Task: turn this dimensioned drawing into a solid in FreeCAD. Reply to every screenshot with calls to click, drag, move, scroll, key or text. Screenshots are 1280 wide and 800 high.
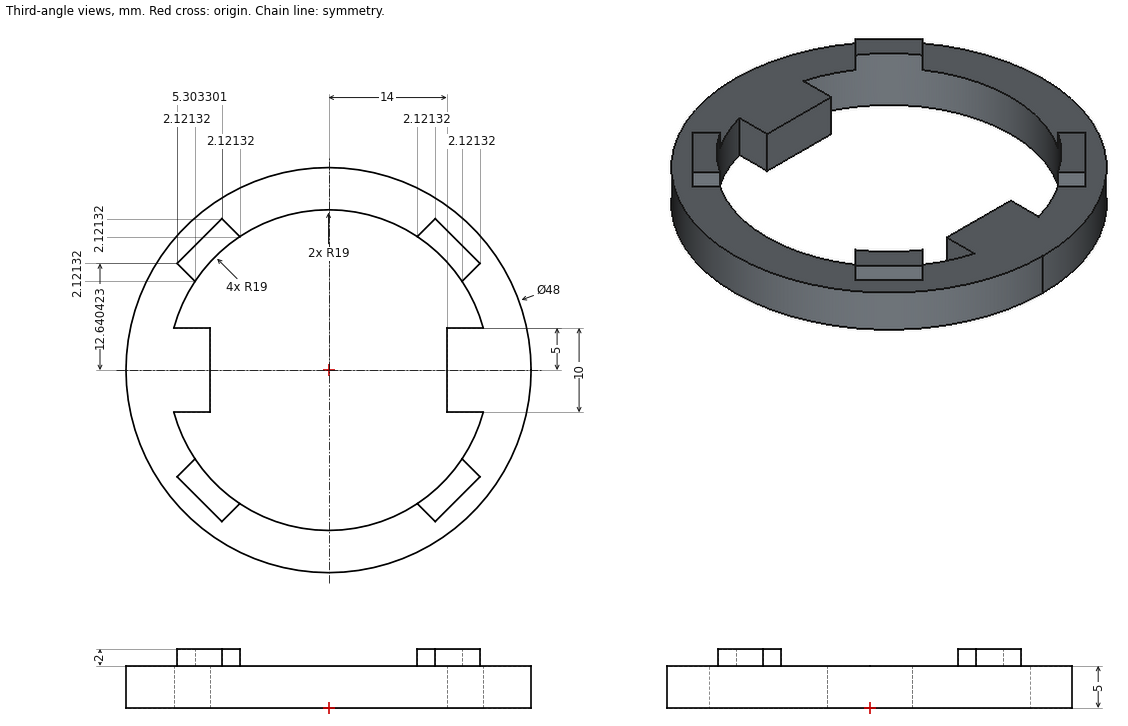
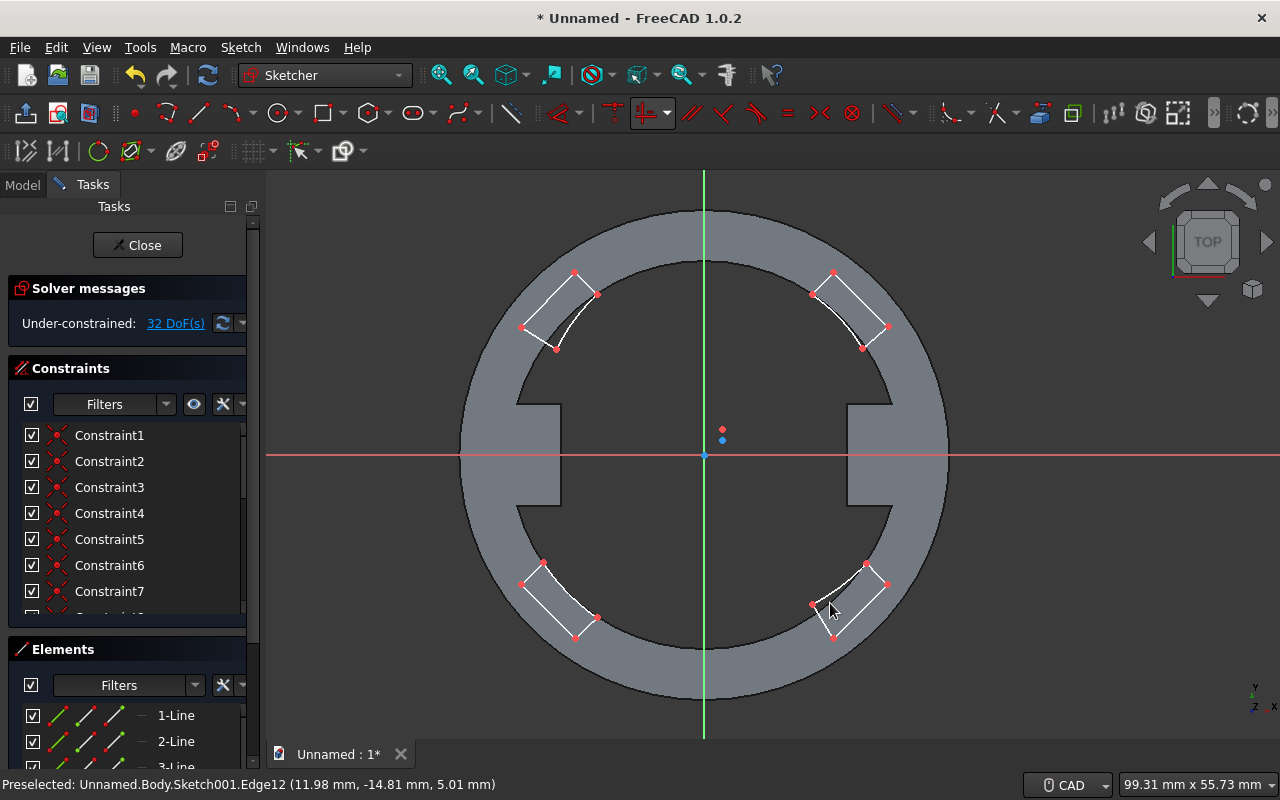
click(583, 309)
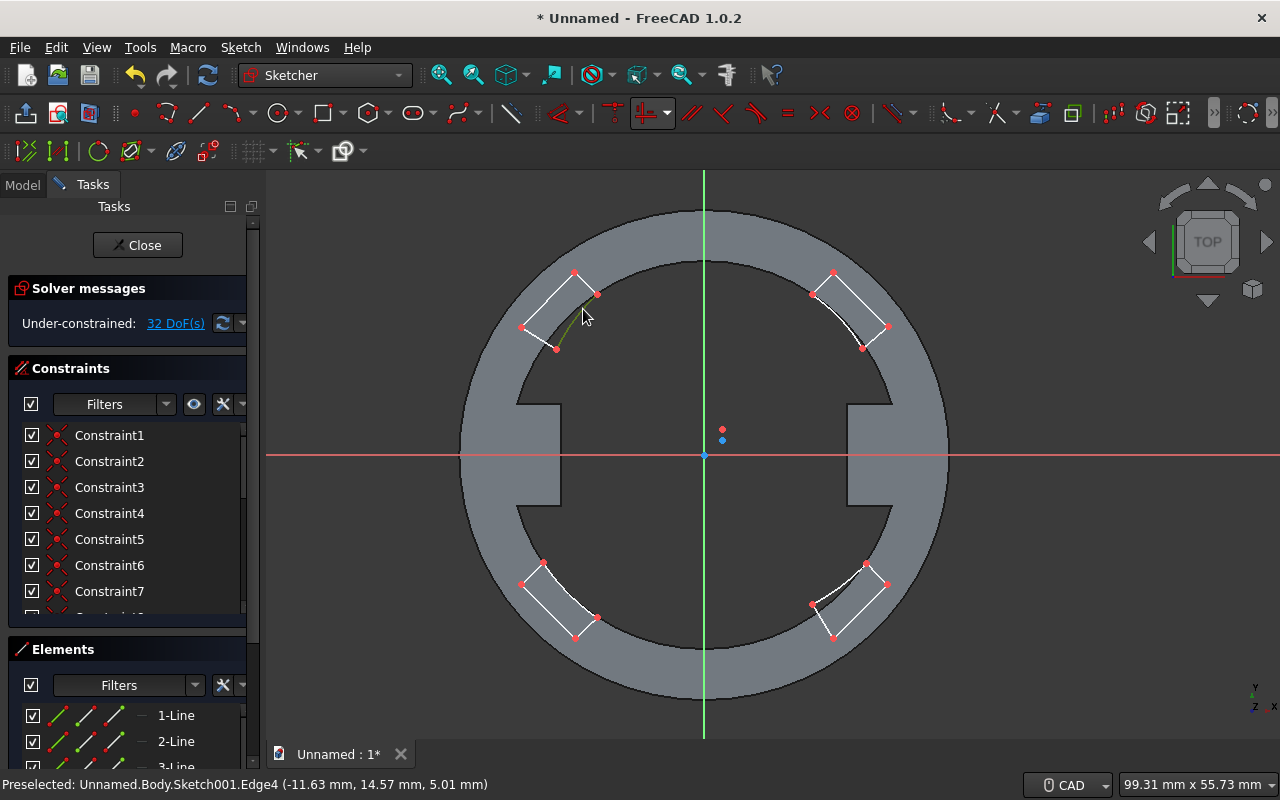
click(557, 581)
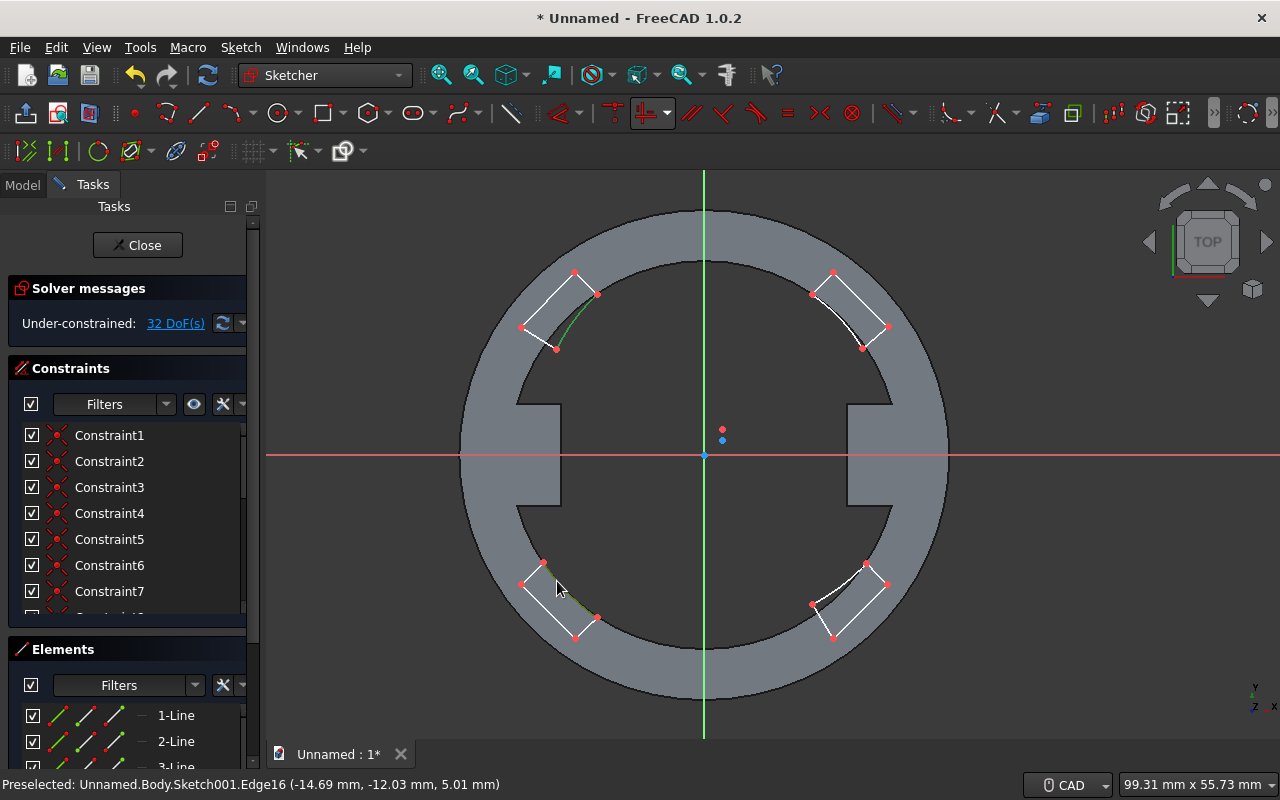
key(c)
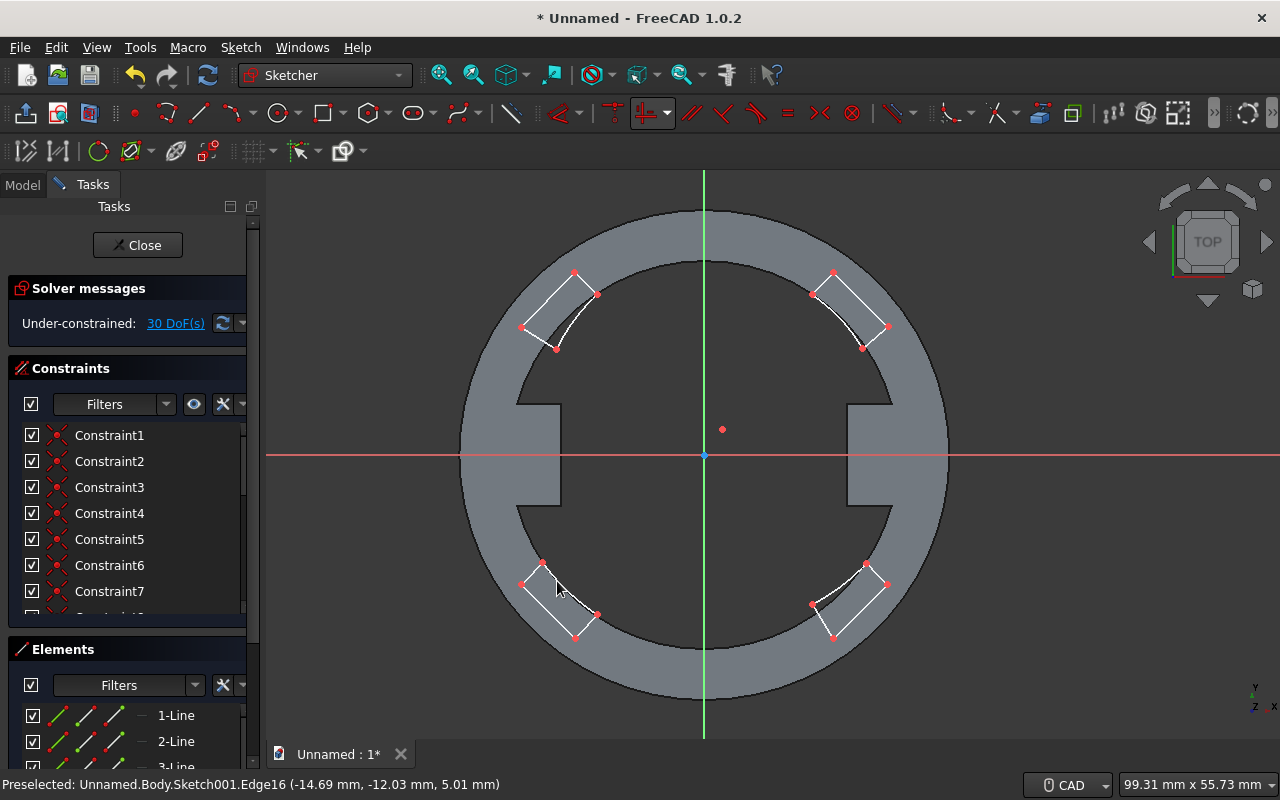
drag(694, 420, 732, 465)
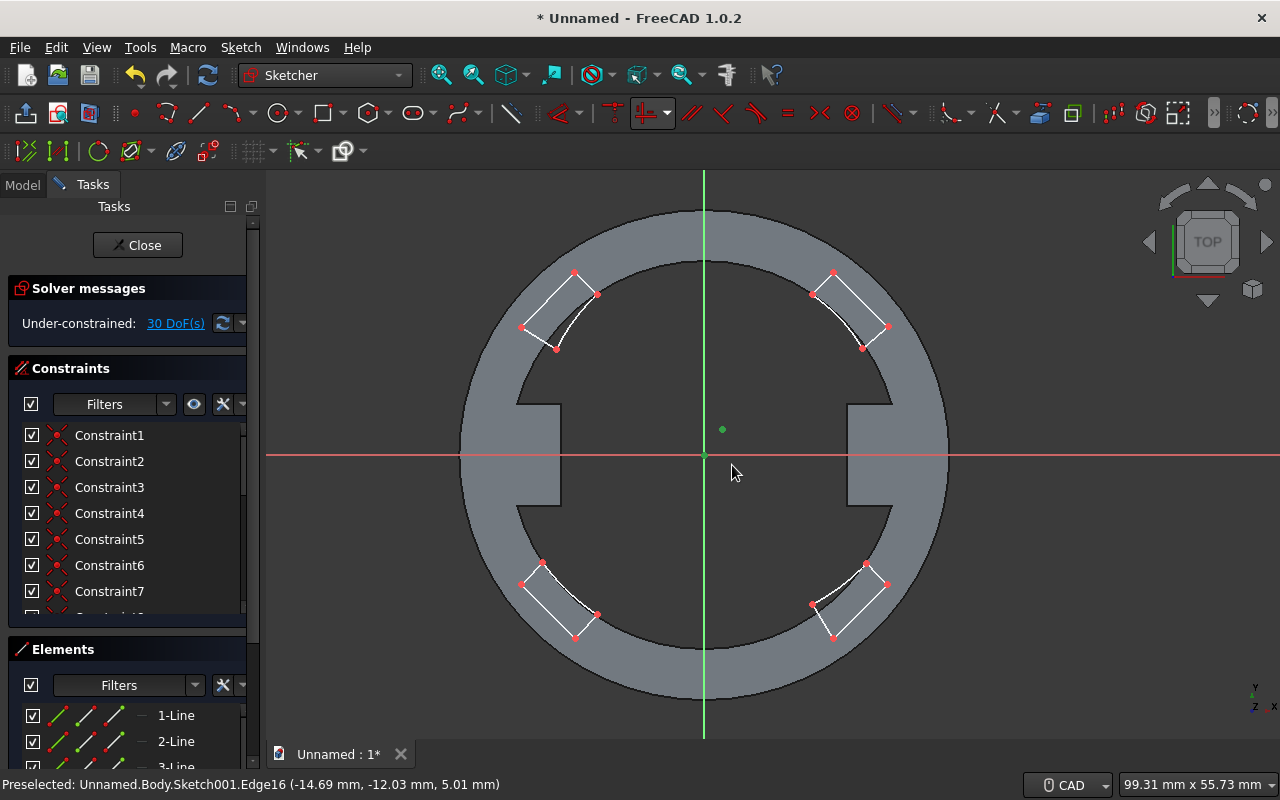
click(614, 114)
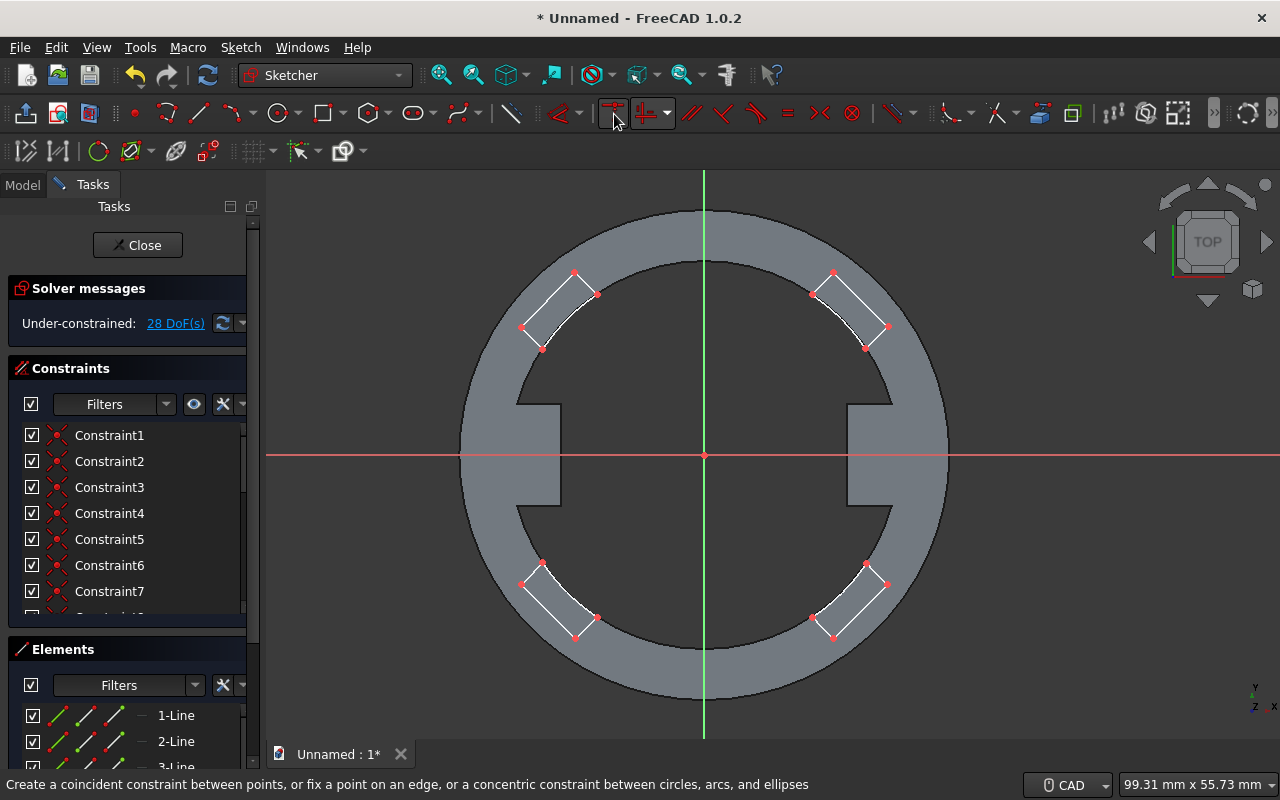
click(579, 309)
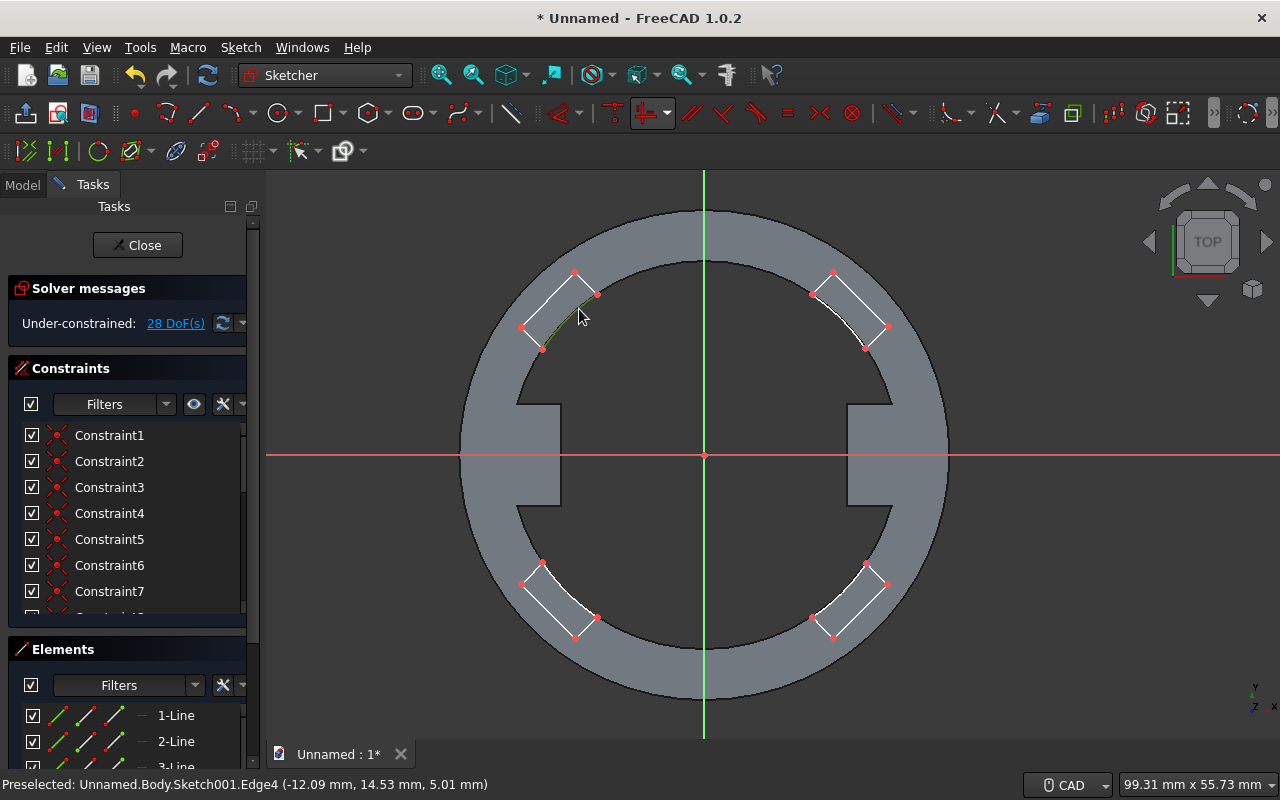
click(852, 331)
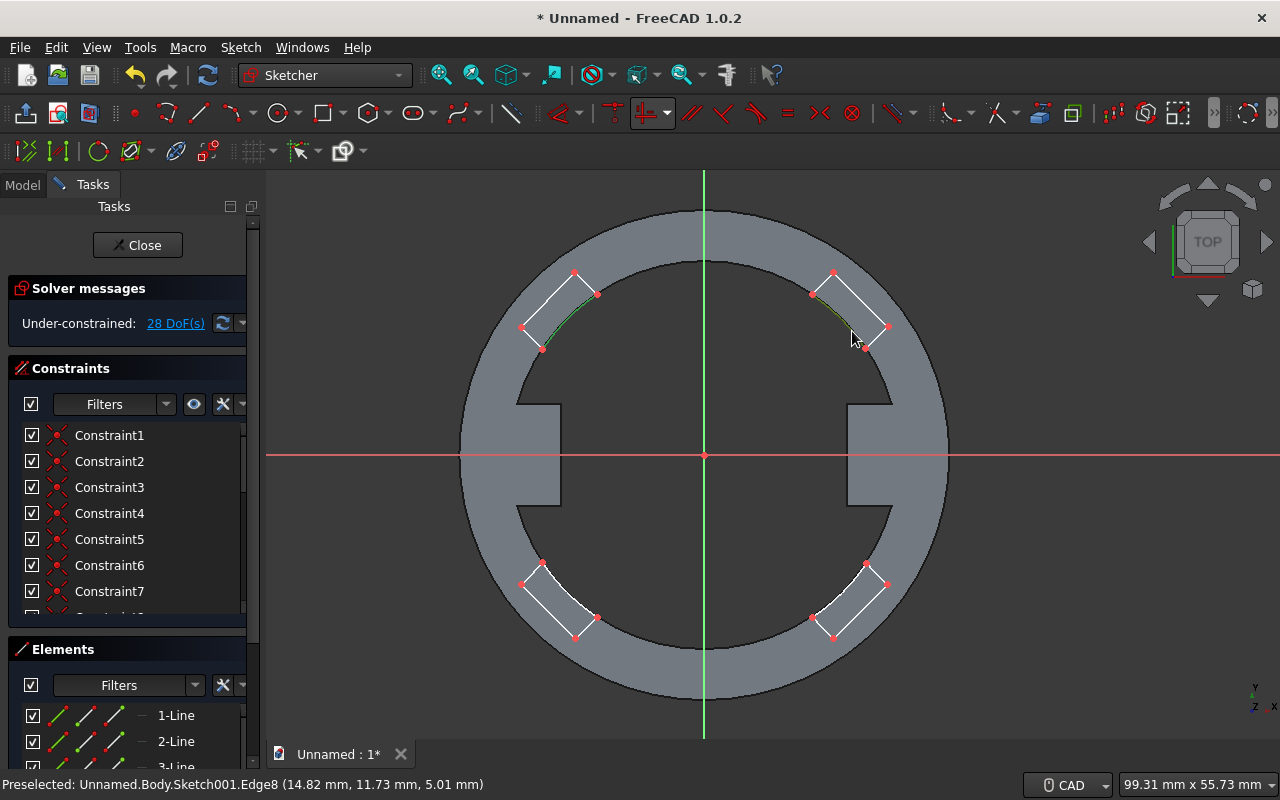
click(831, 603)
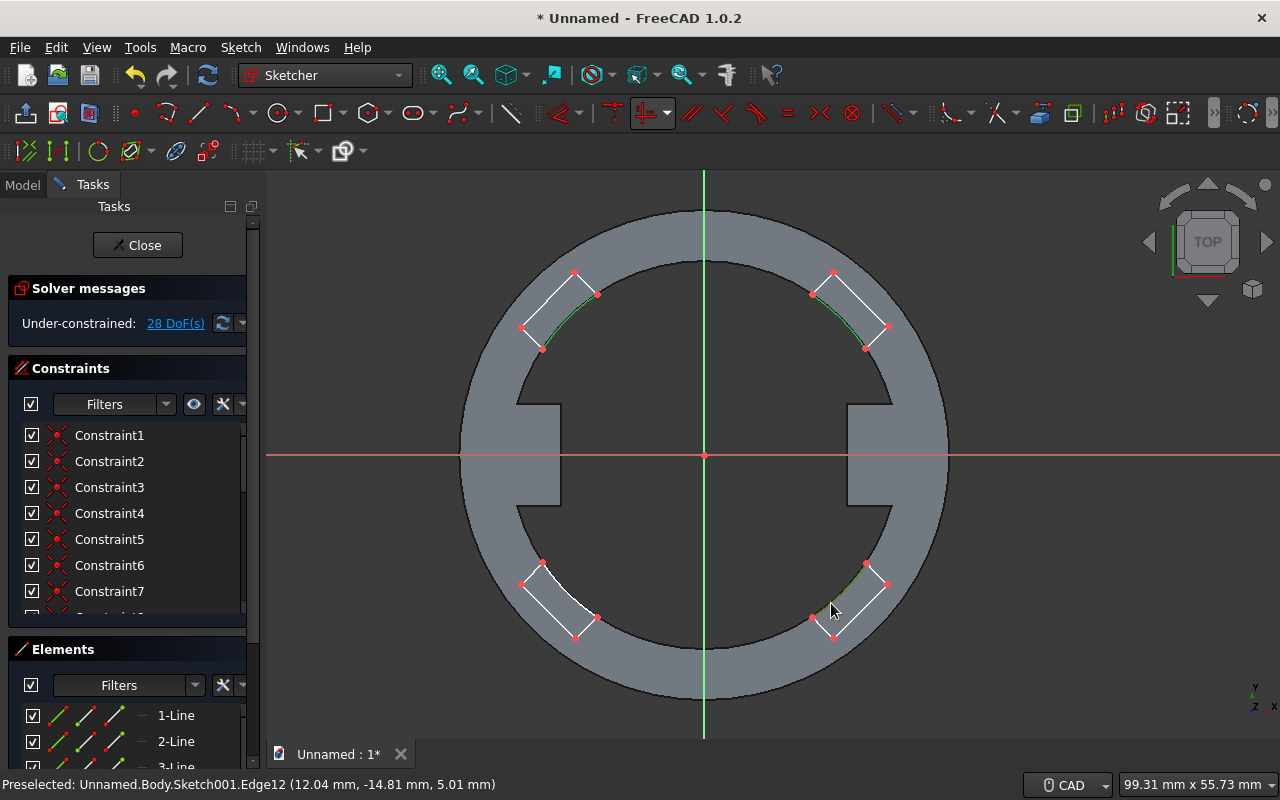
click(557, 581)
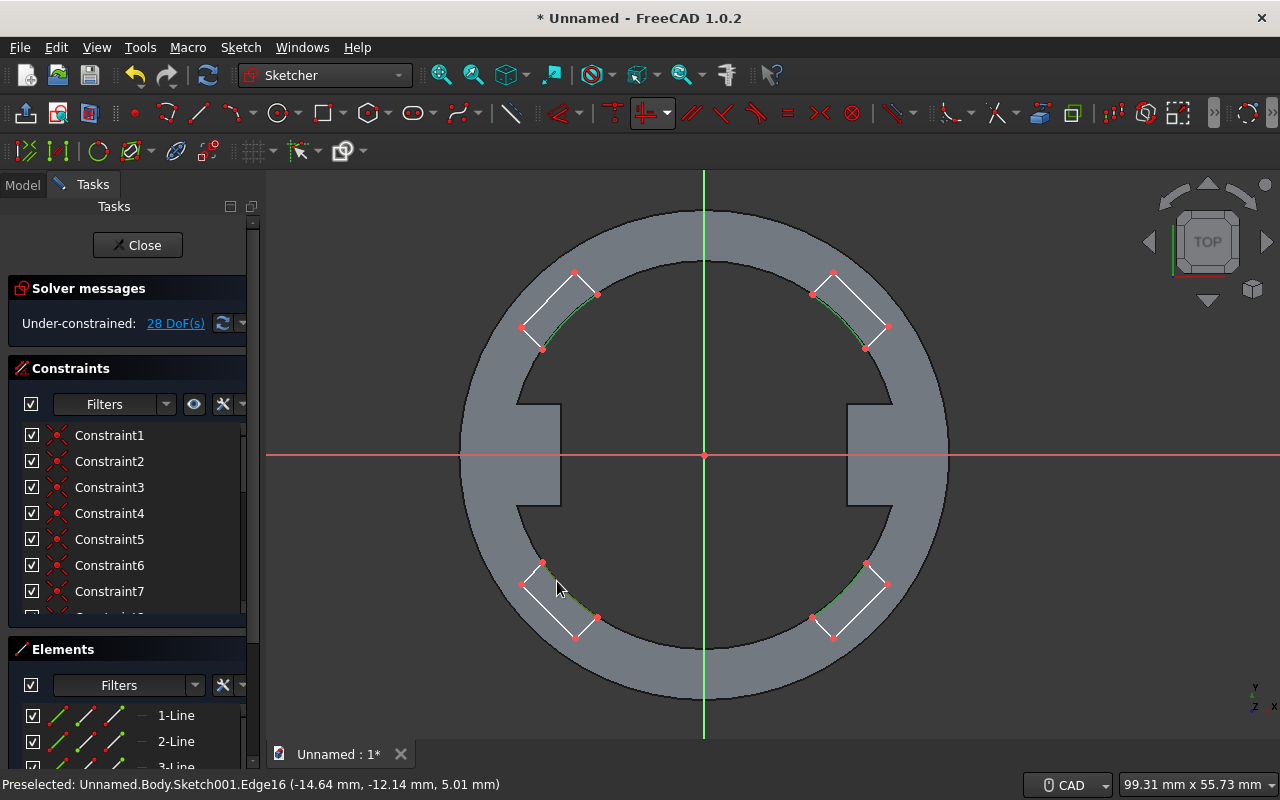
key(e)